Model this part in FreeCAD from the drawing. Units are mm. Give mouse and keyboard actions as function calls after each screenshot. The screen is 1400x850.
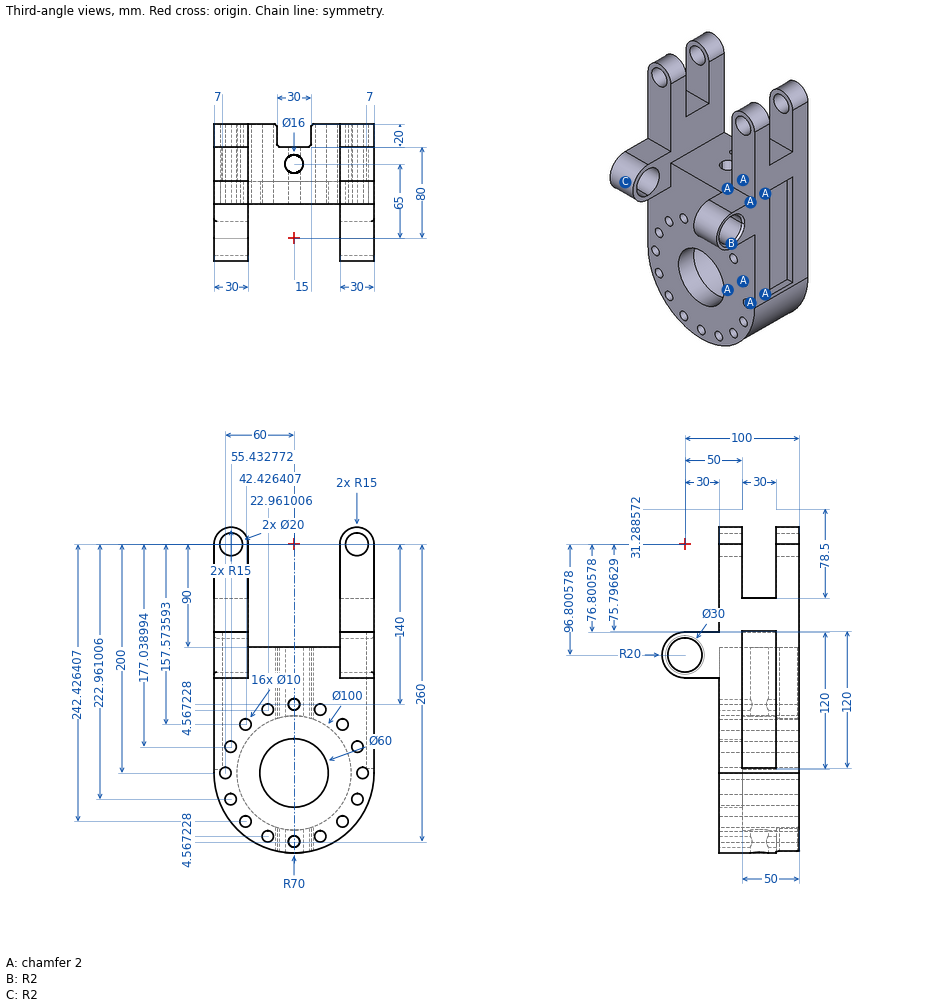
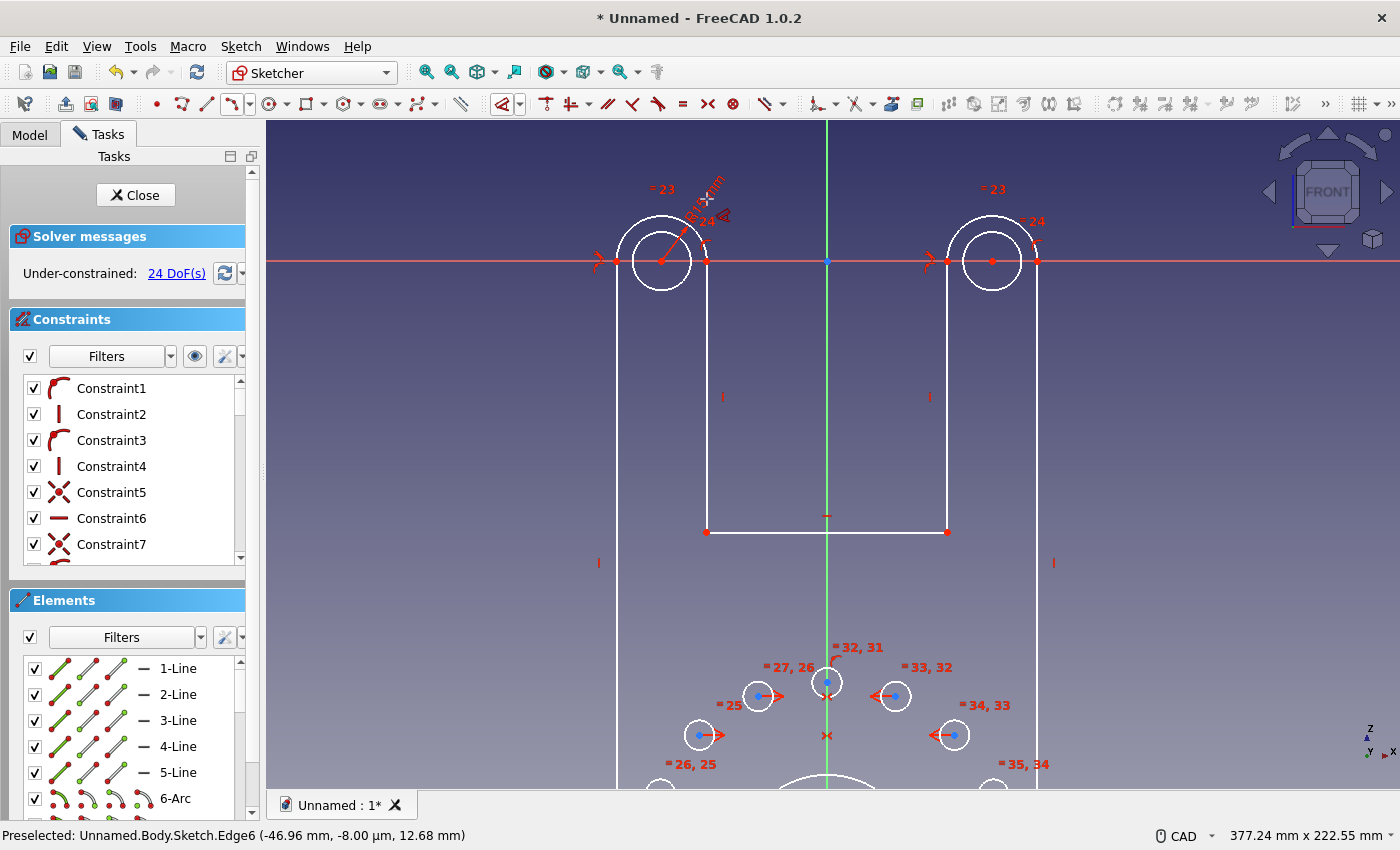
scroll(688, 223, down, 3)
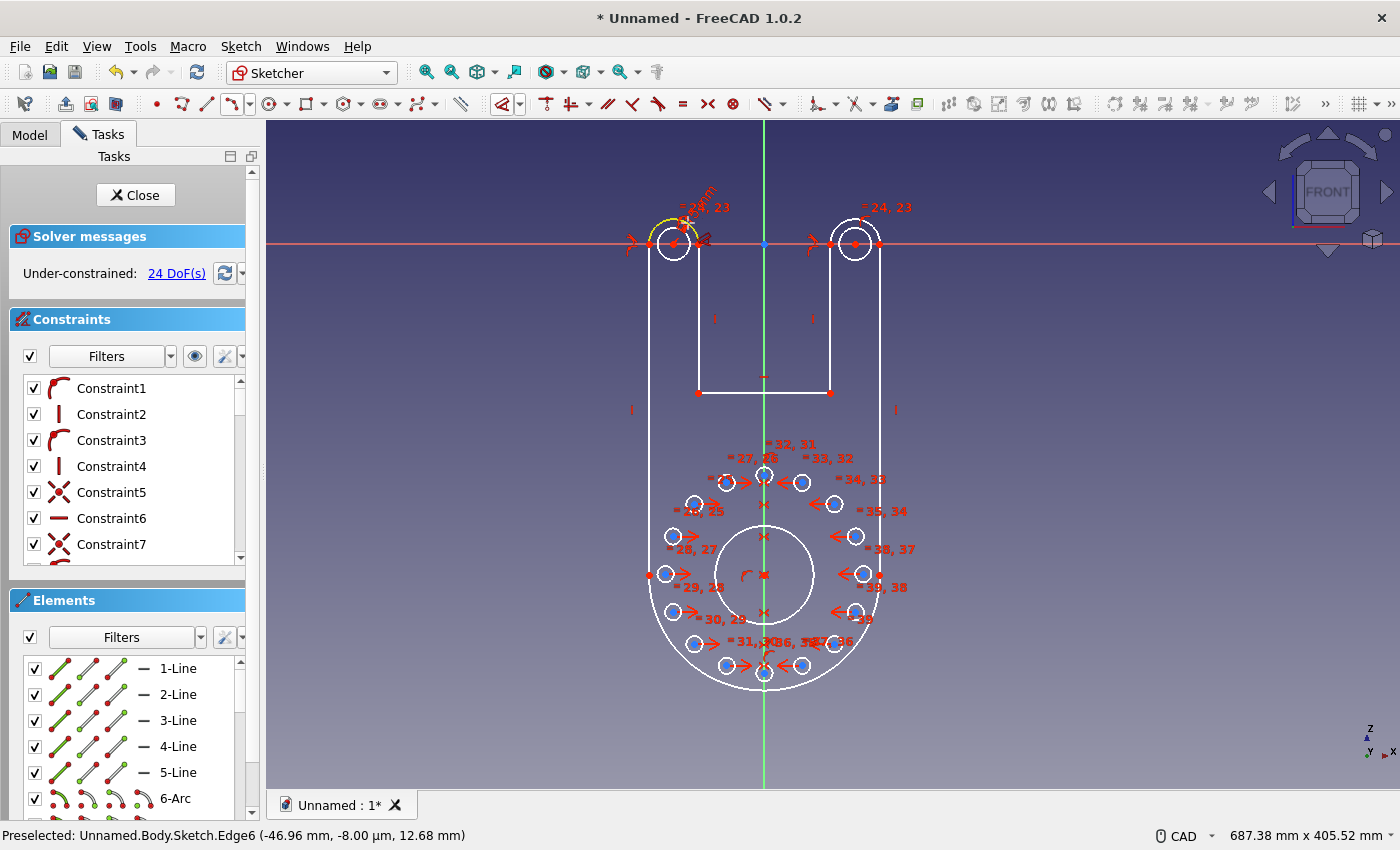
click(697, 669)
click(678, 695)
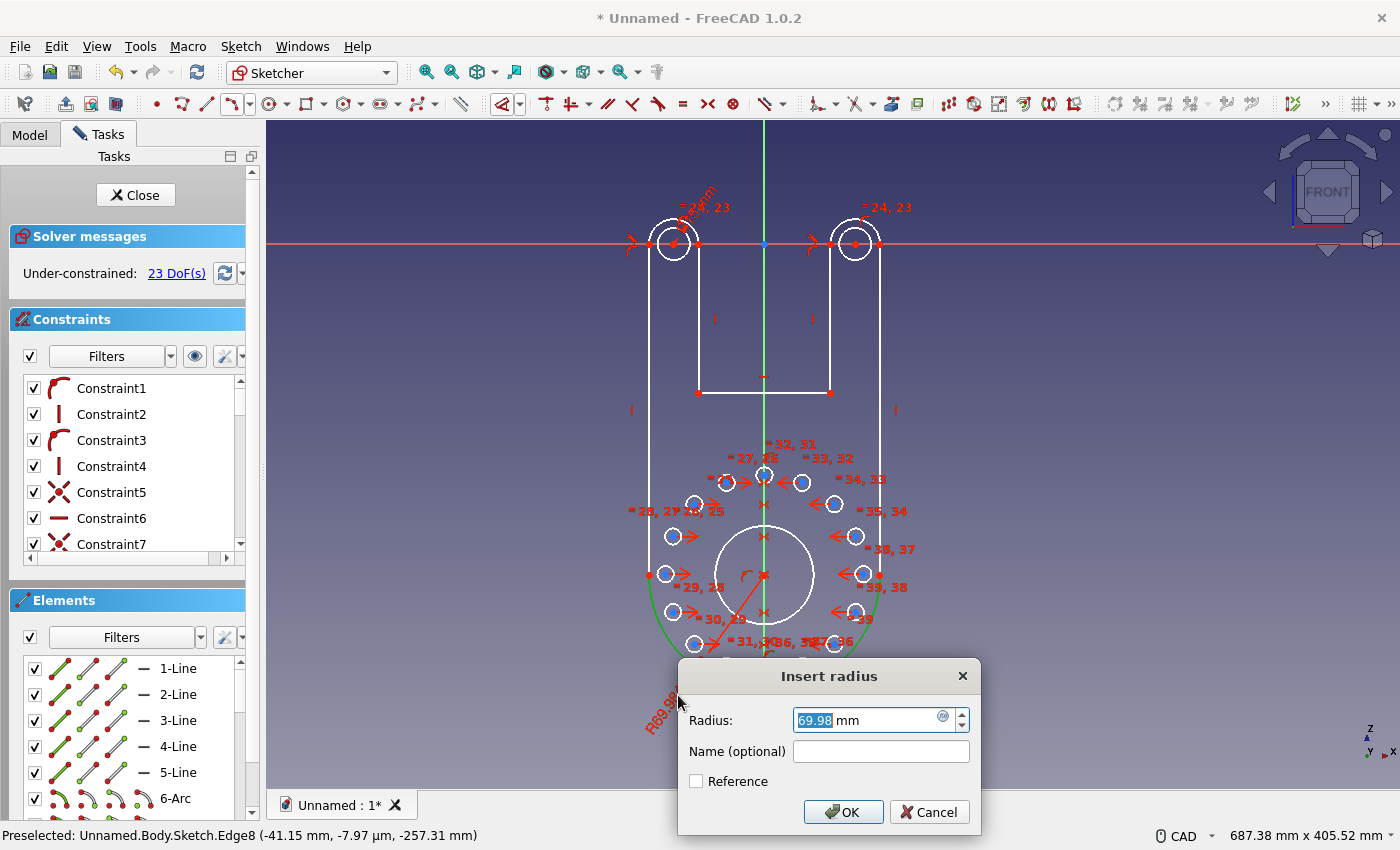
text(70)
key(Return)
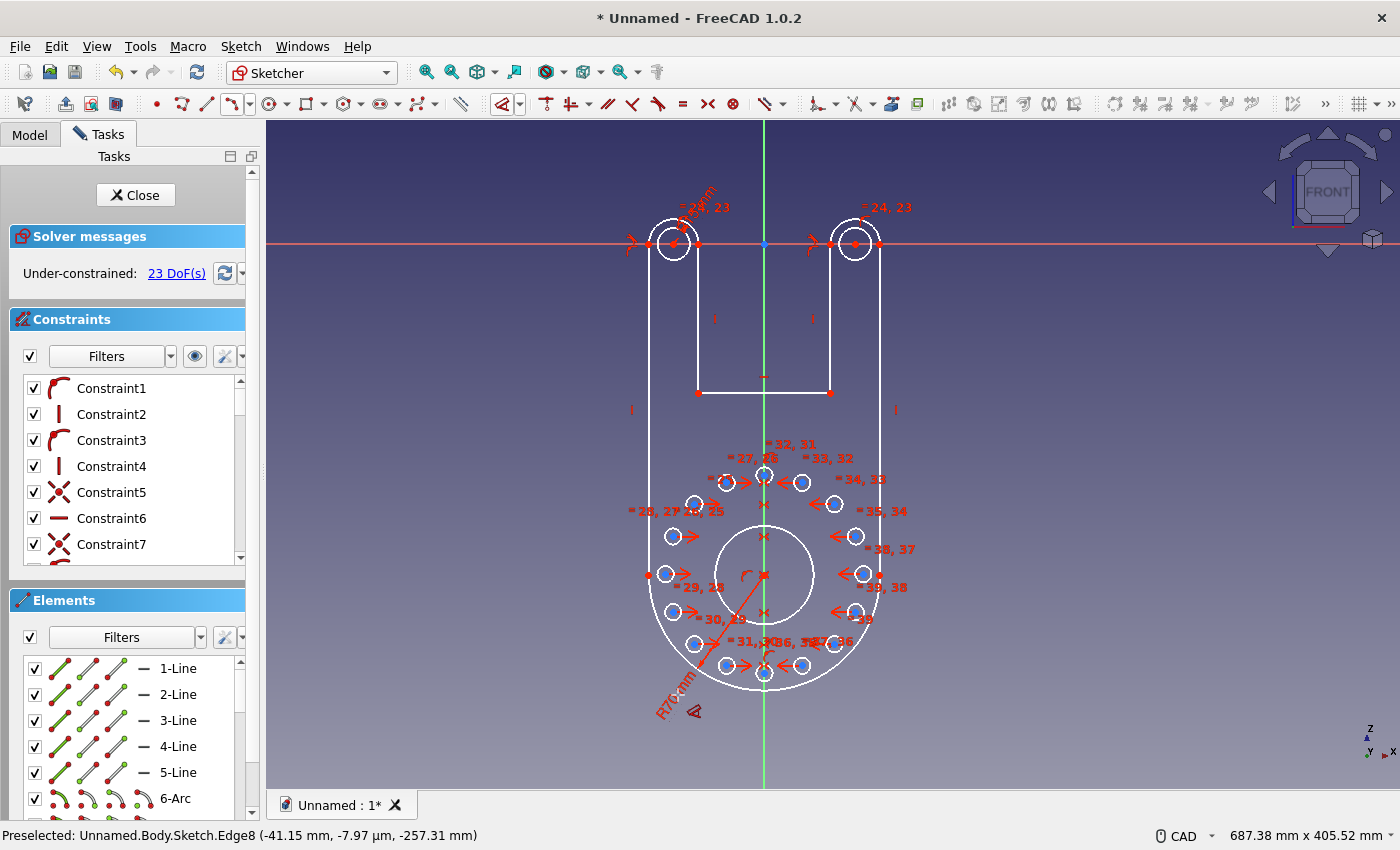
click(662, 255)
click(682, 291)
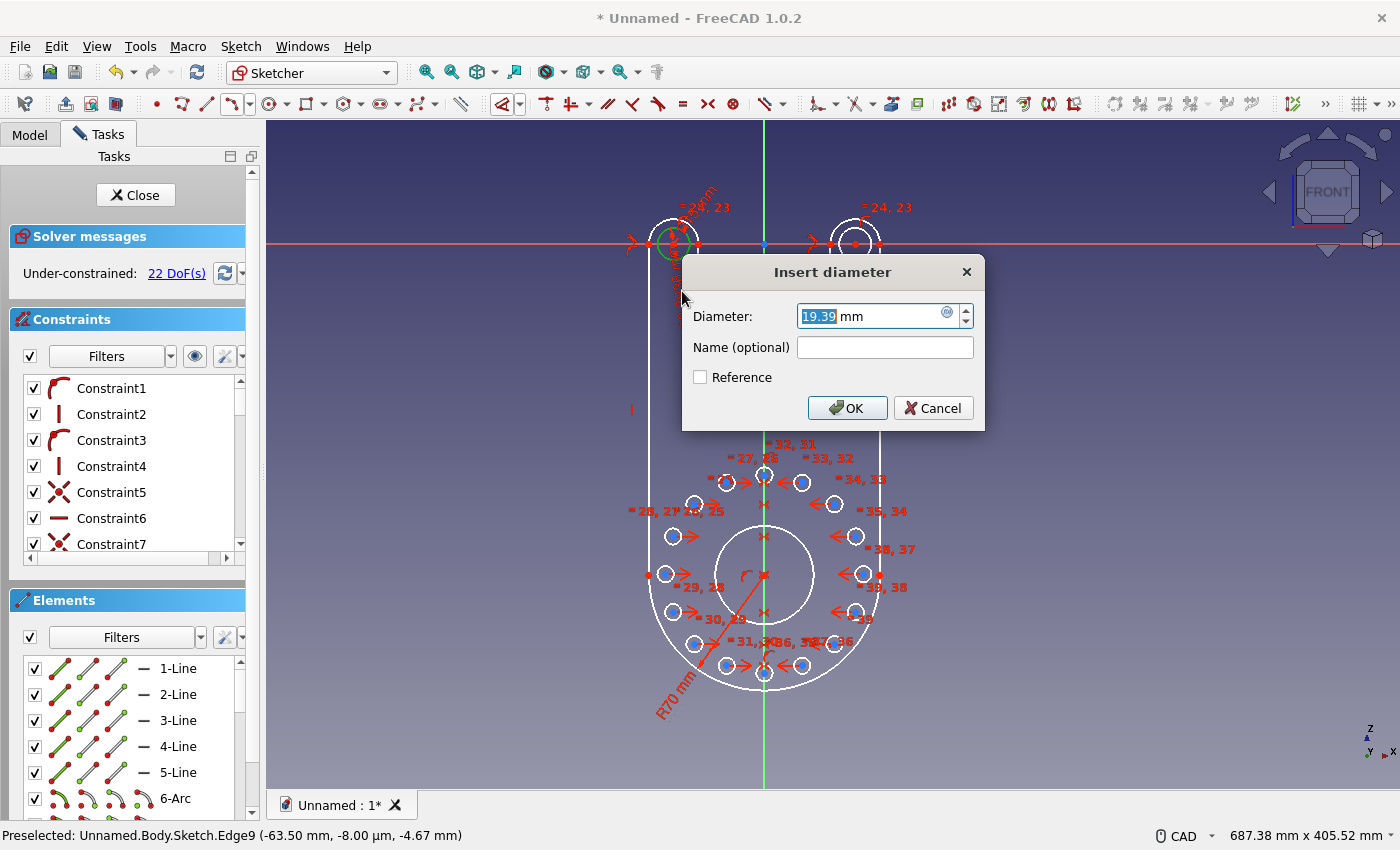
text(20)
key(Return)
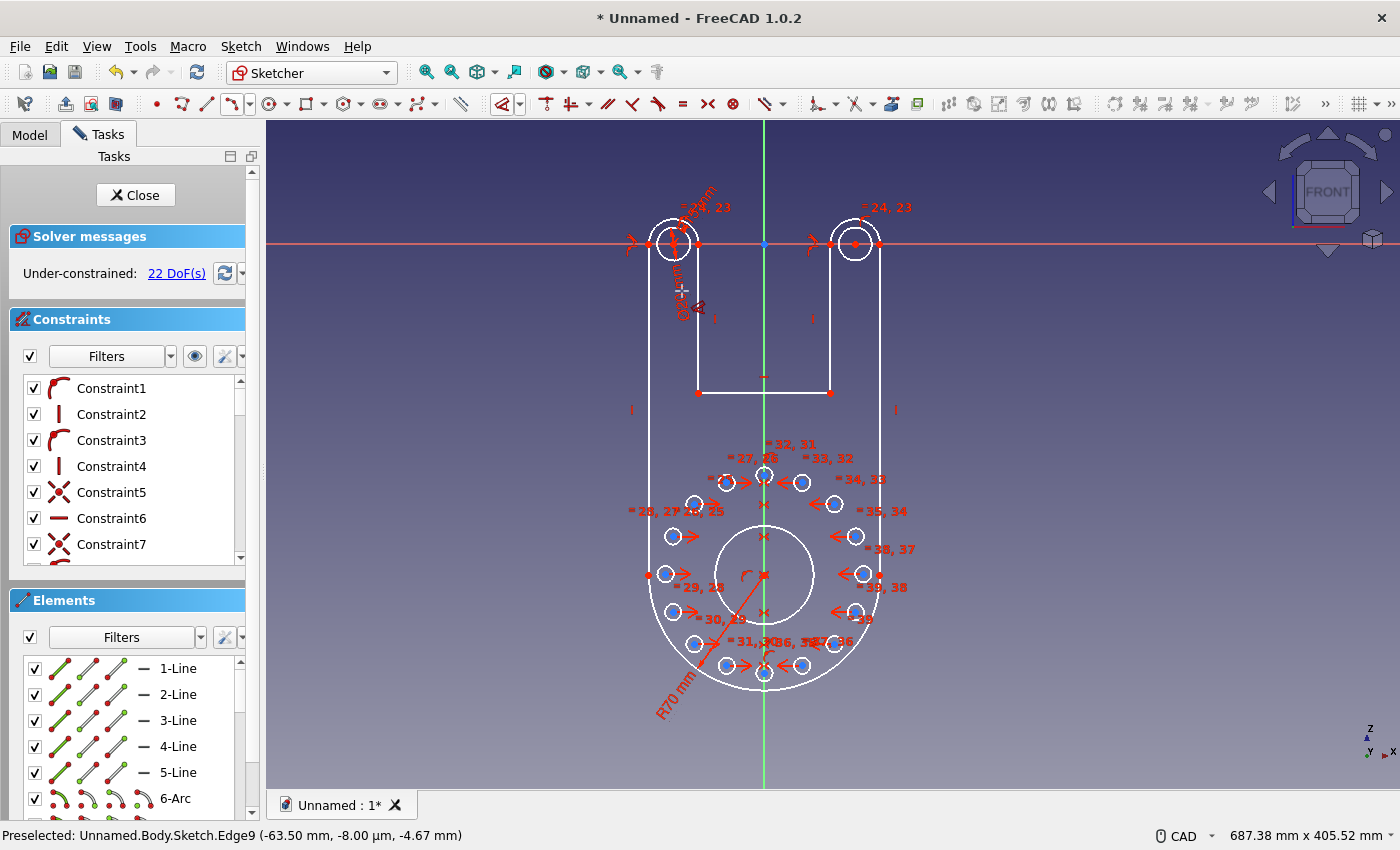
scroll(700, 510, up, 5)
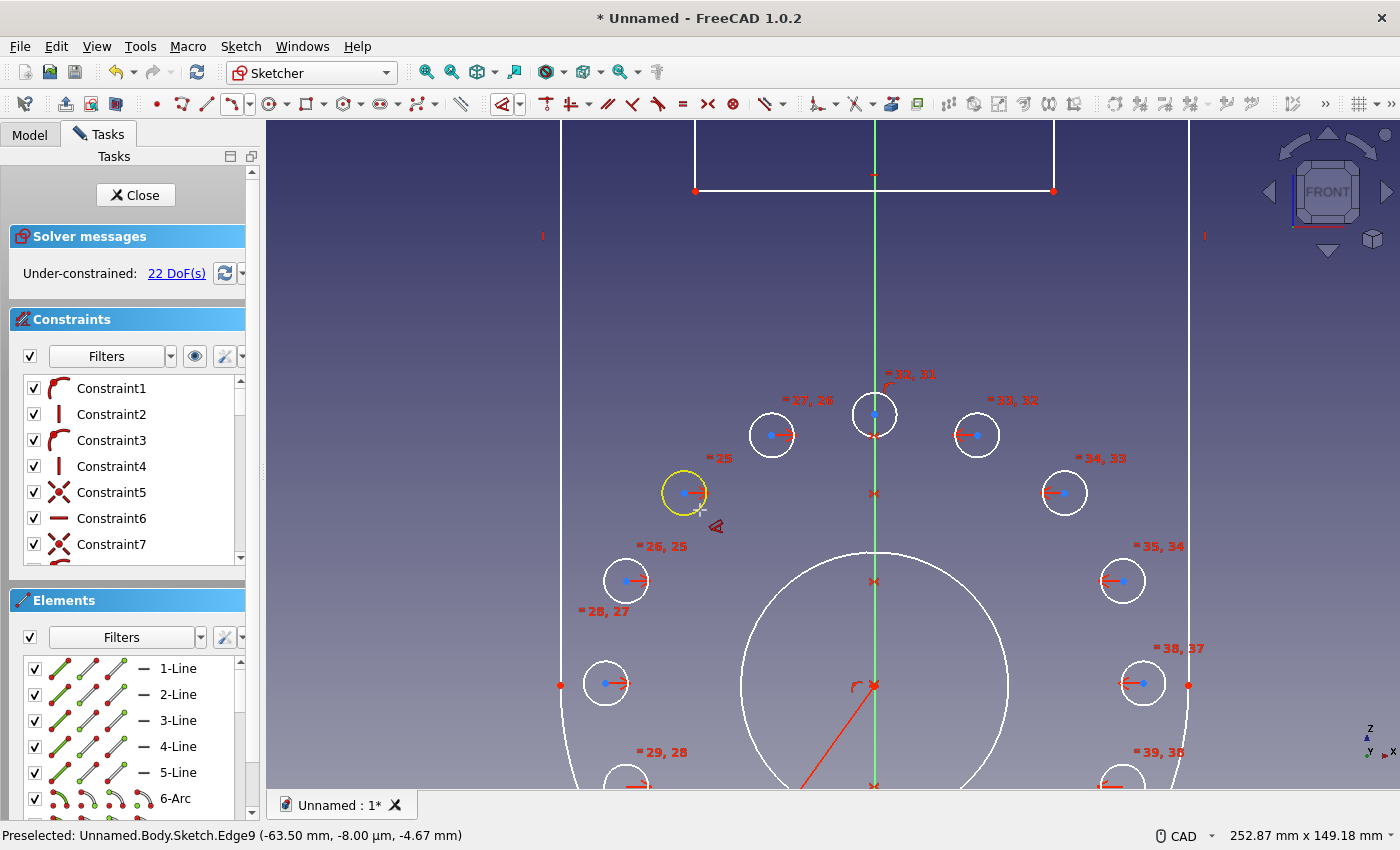
click(700, 509)
click(723, 532)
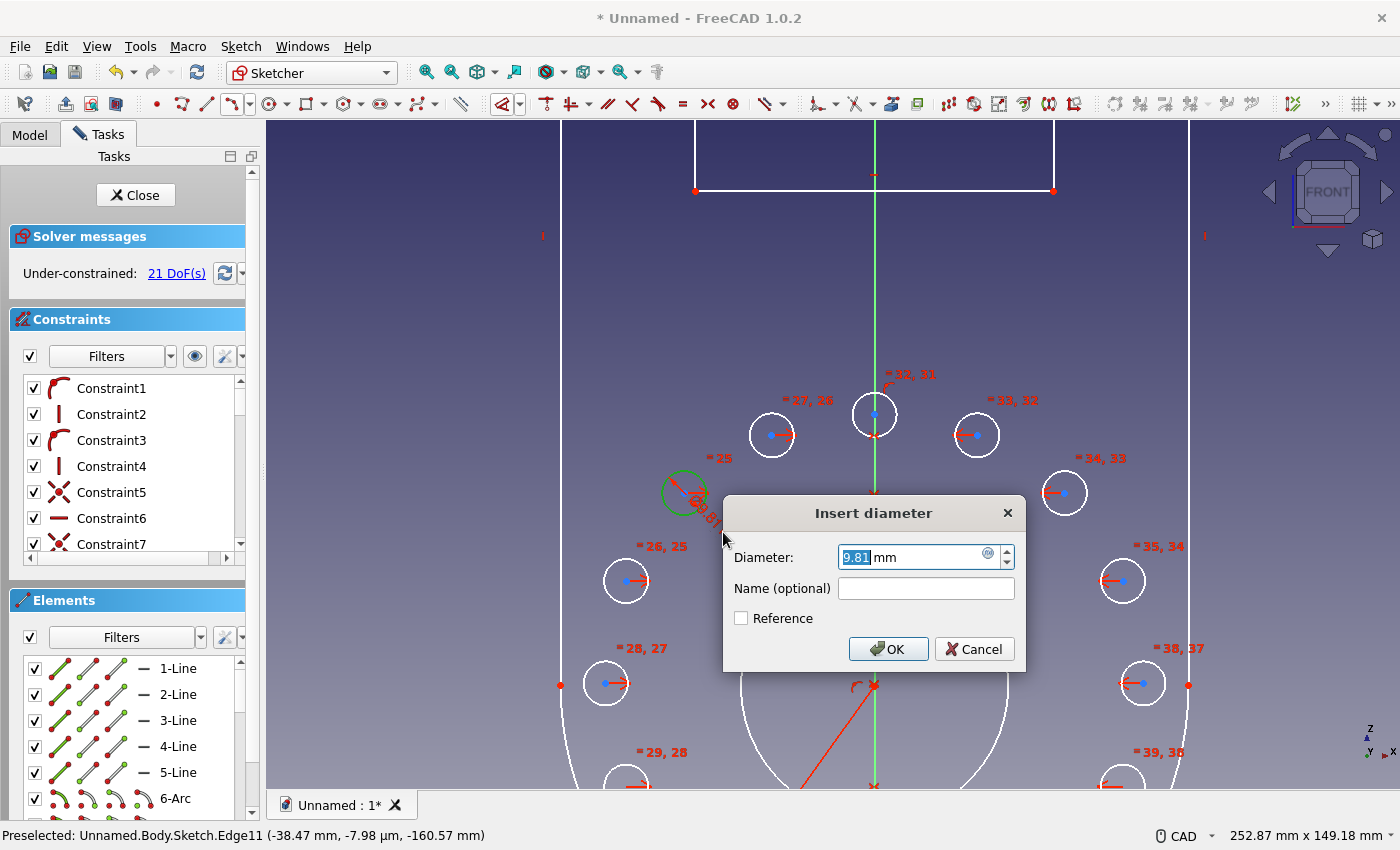
text(10)
key(Return)